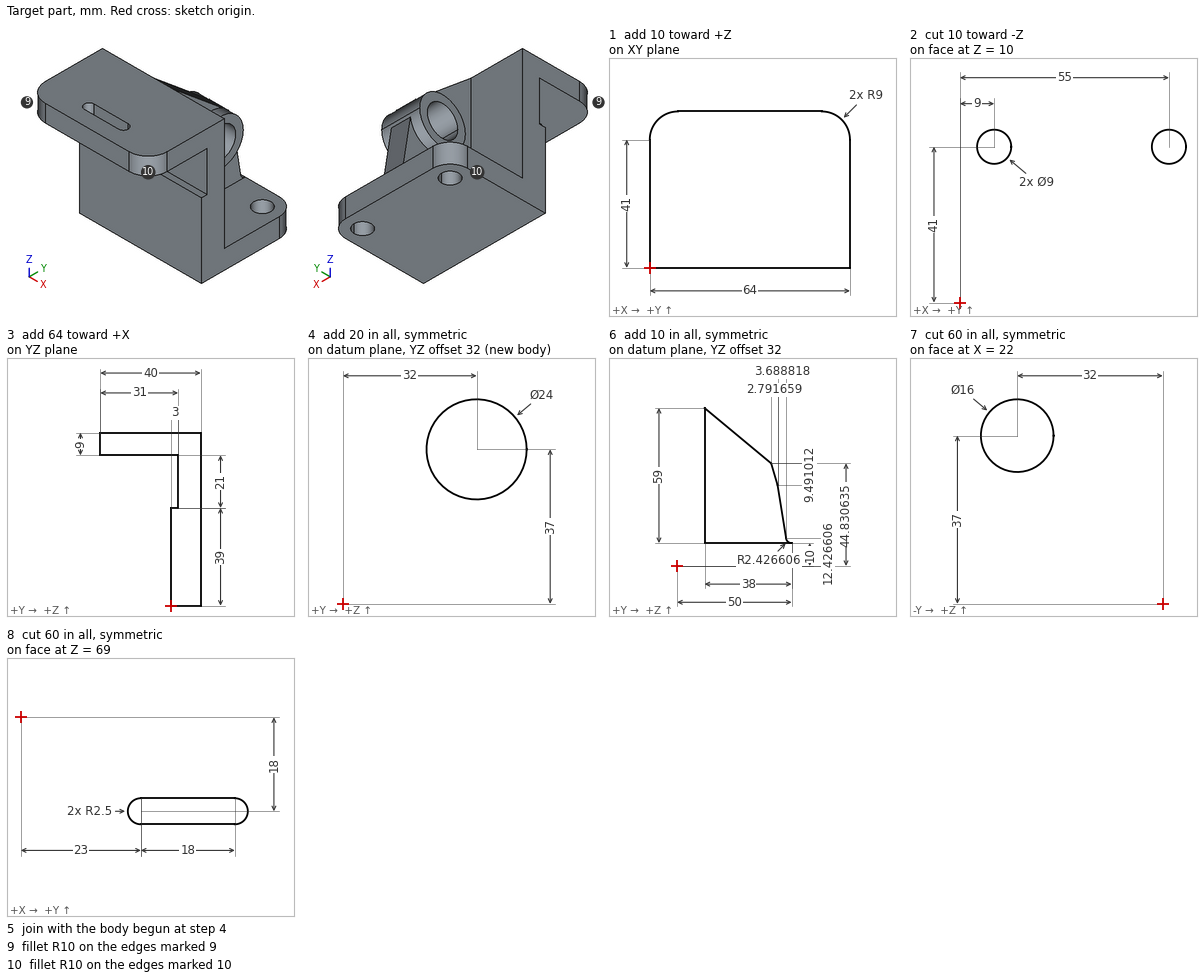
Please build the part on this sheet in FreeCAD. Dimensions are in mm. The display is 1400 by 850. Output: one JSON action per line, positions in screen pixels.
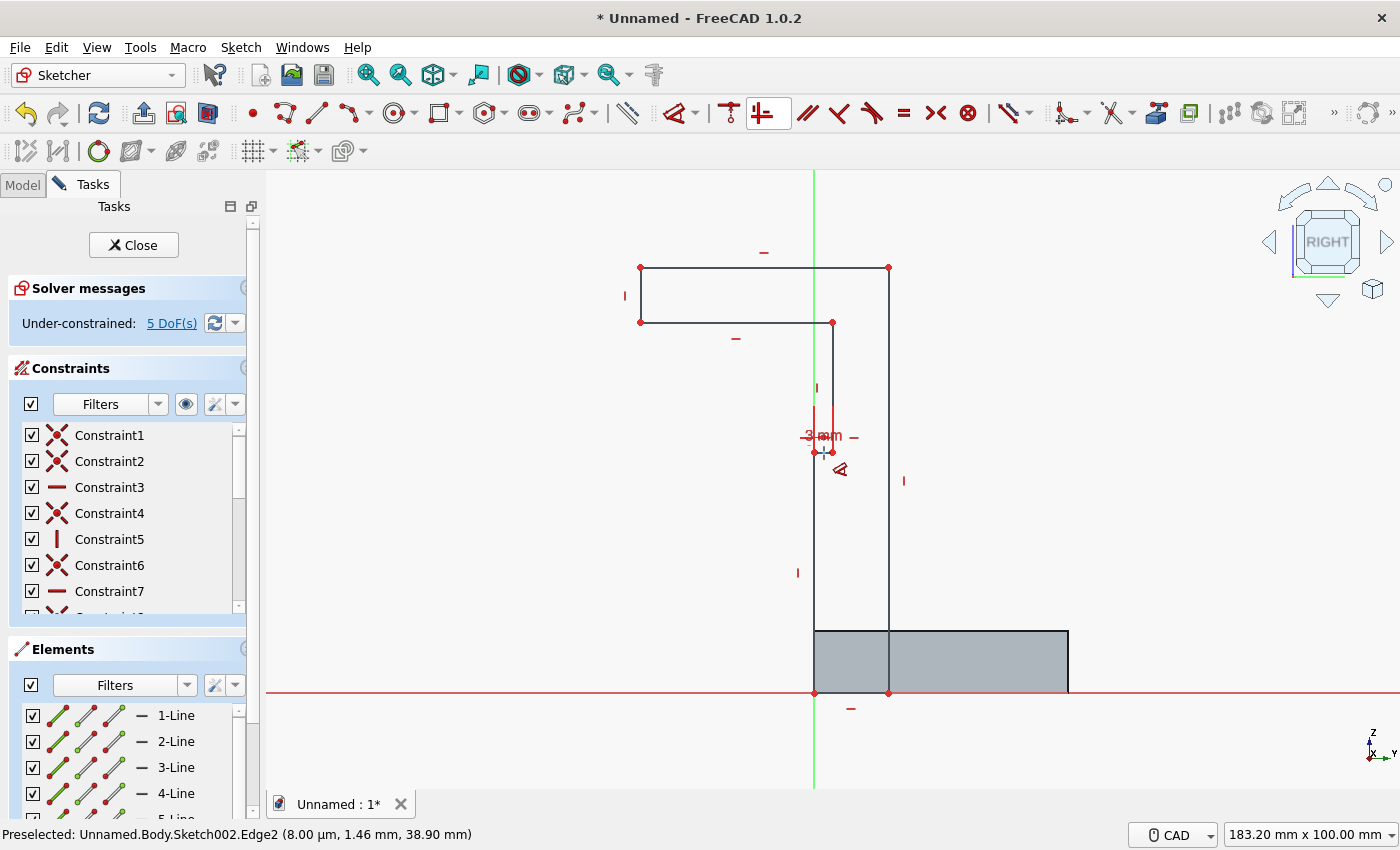
{"action": "left_click", "coordinate": [641, 306]}
{"action": "left_click", "coordinate": [607, 295]}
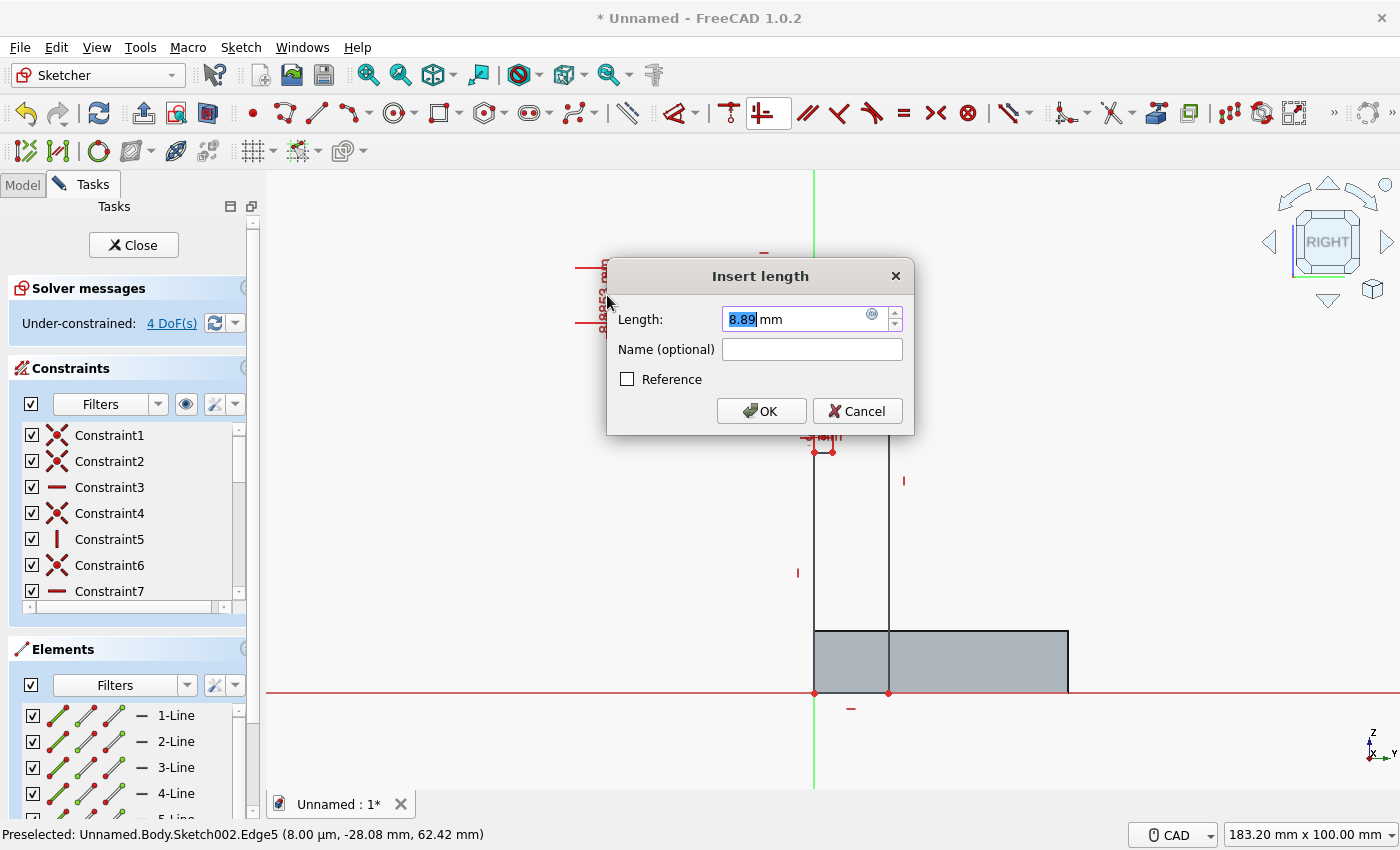
{"action": "type", "text": "9"}
{"action": "key", "text": "Return"}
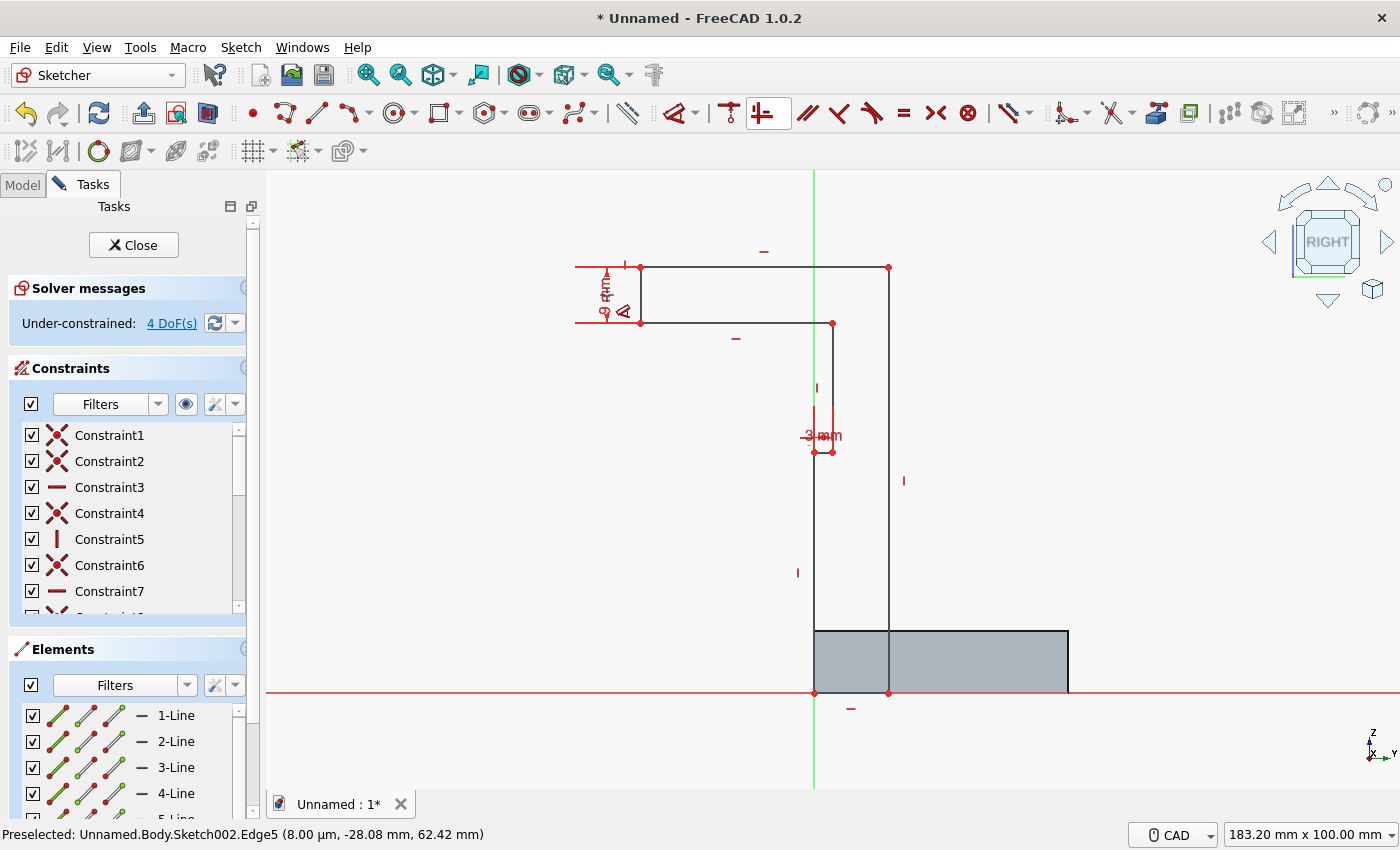
{"action": "left_click", "coordinate": [814, 621]}
{"action": "left_click", "coordinate": [848, 573]}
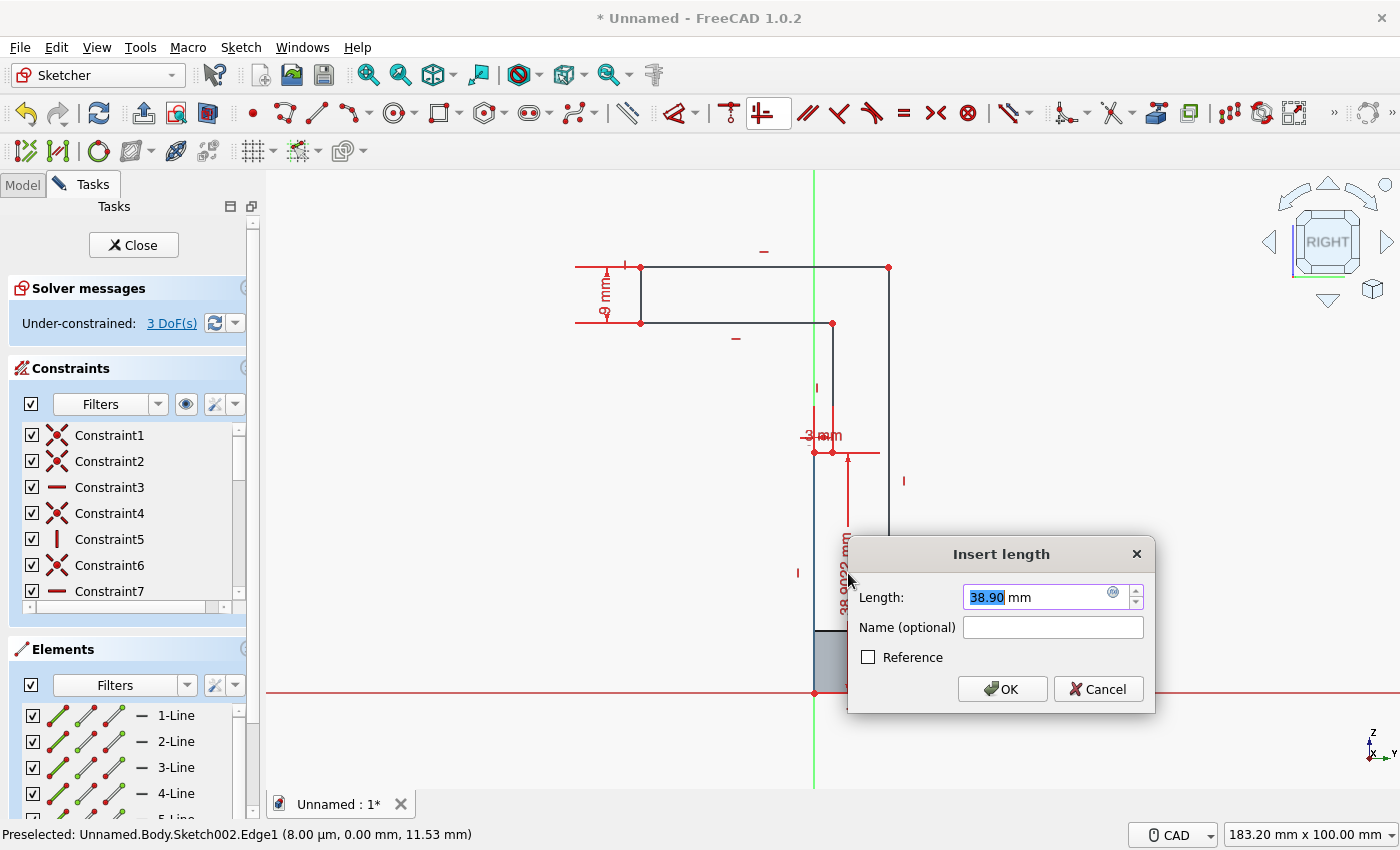
{"action": "type", "text": "39"}
{"action": "key", "text": "Return"}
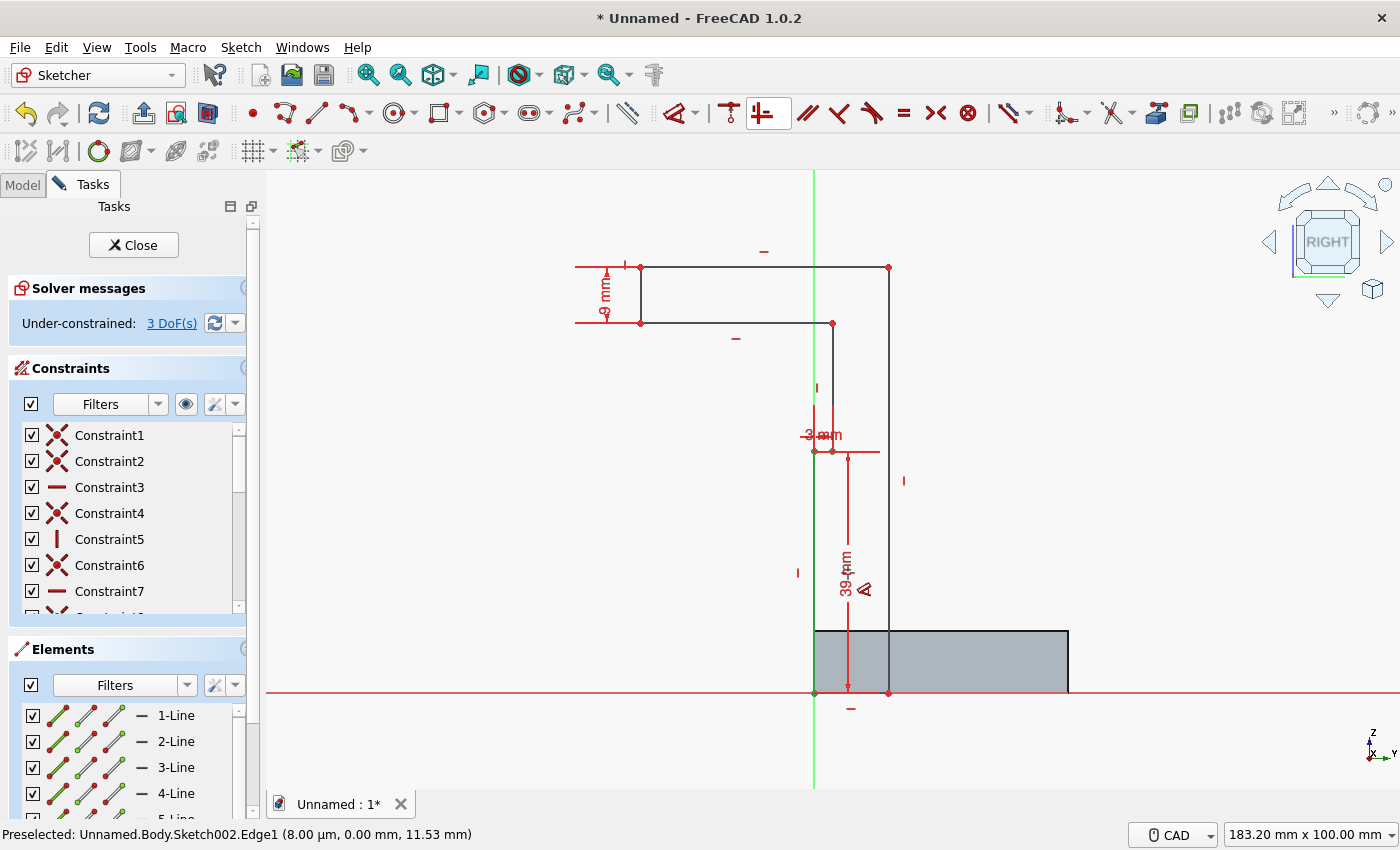
{"action": "left_click", "coordinate": [833, 413]}
{"action": "left_click", "coordinate": [867, 388]}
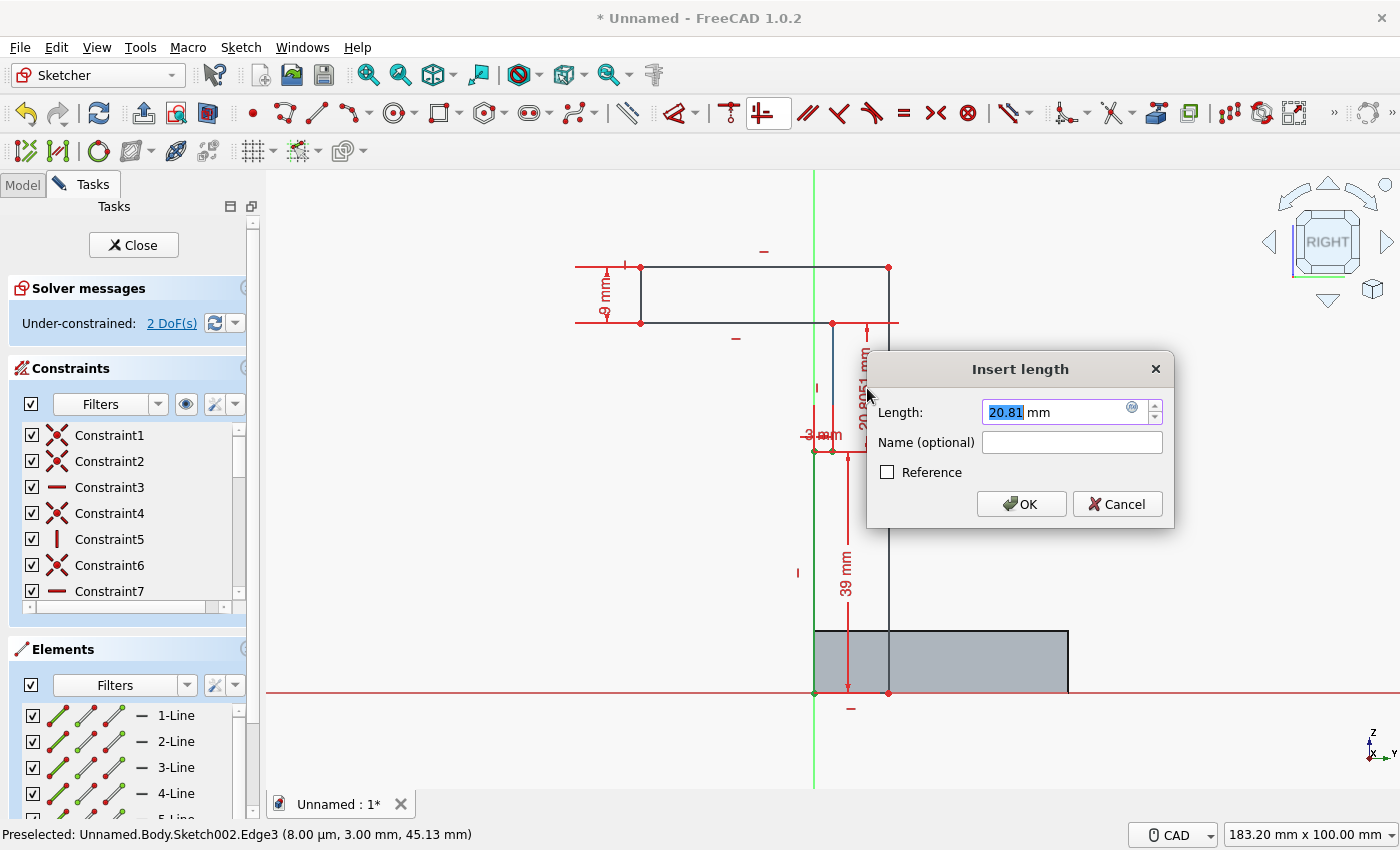
{"action": "type", "text": "21"}
{"action": "key", "text": "Return"}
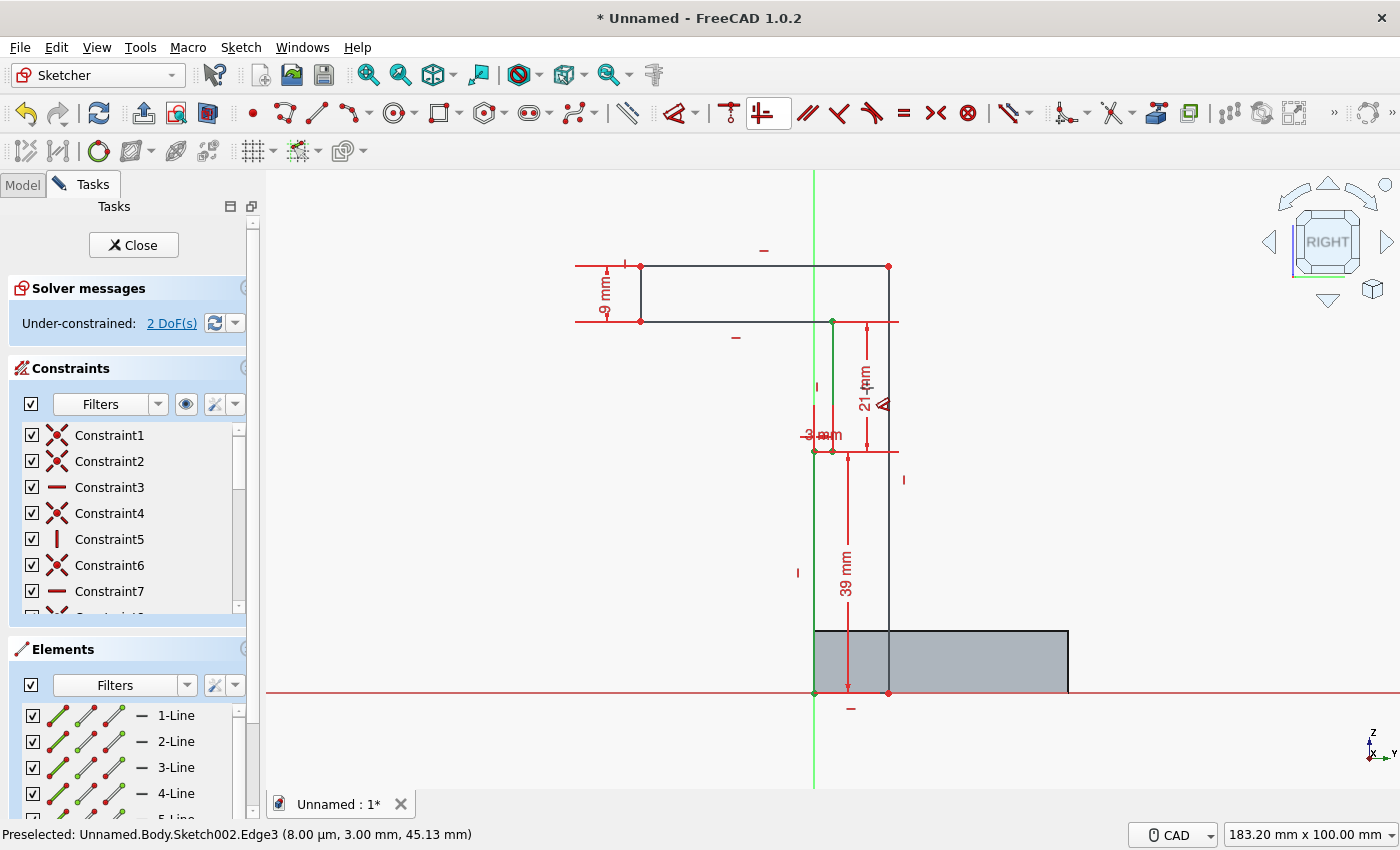
{"action": "left_click", "coordinate": [775, 322]}
{"action": "left_click", "coordinate": [737, 288]}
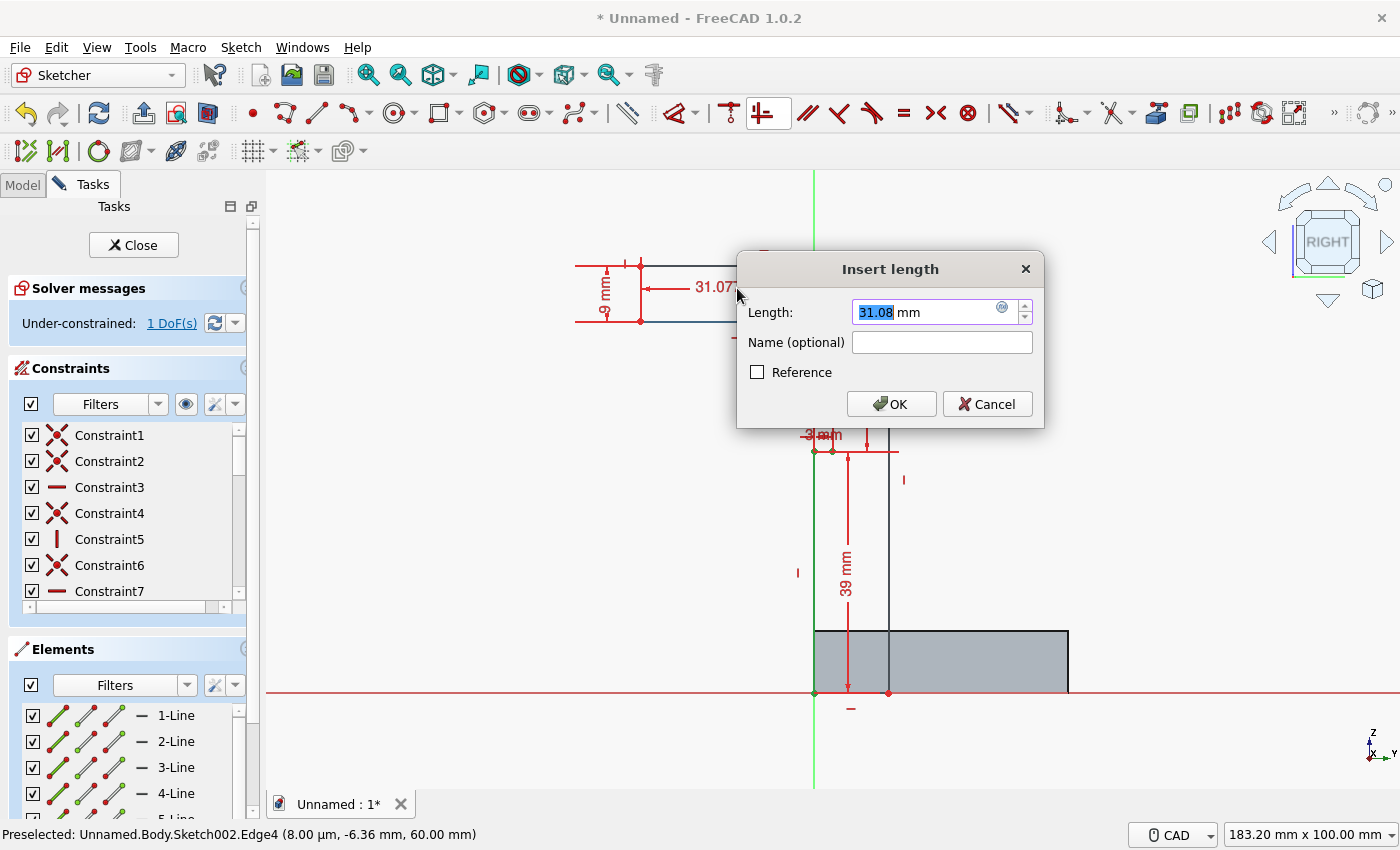
{"action": "type", "text": "31"}
{"action": "key", "text": "Return"}